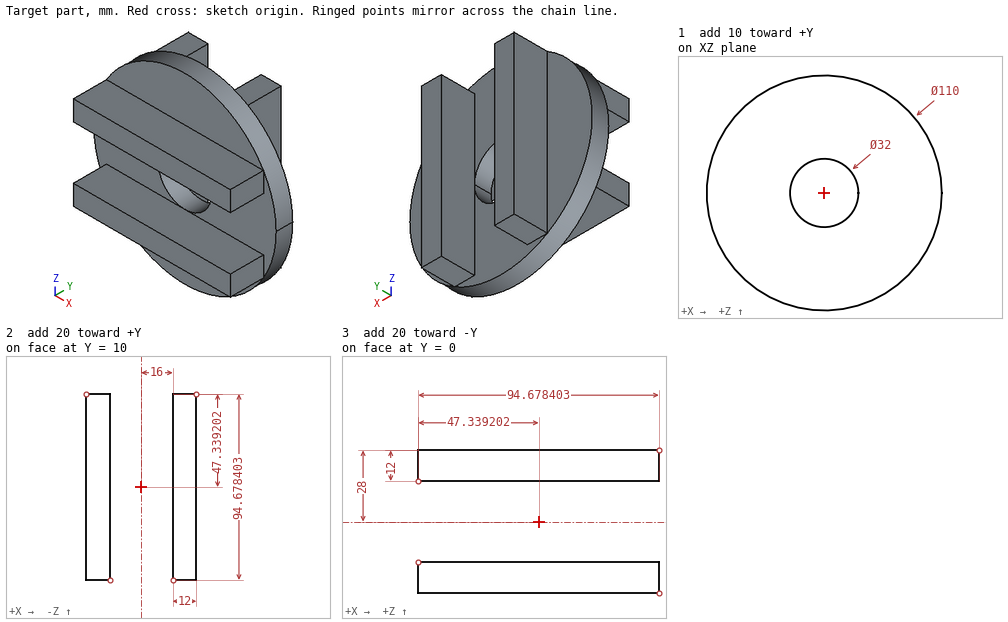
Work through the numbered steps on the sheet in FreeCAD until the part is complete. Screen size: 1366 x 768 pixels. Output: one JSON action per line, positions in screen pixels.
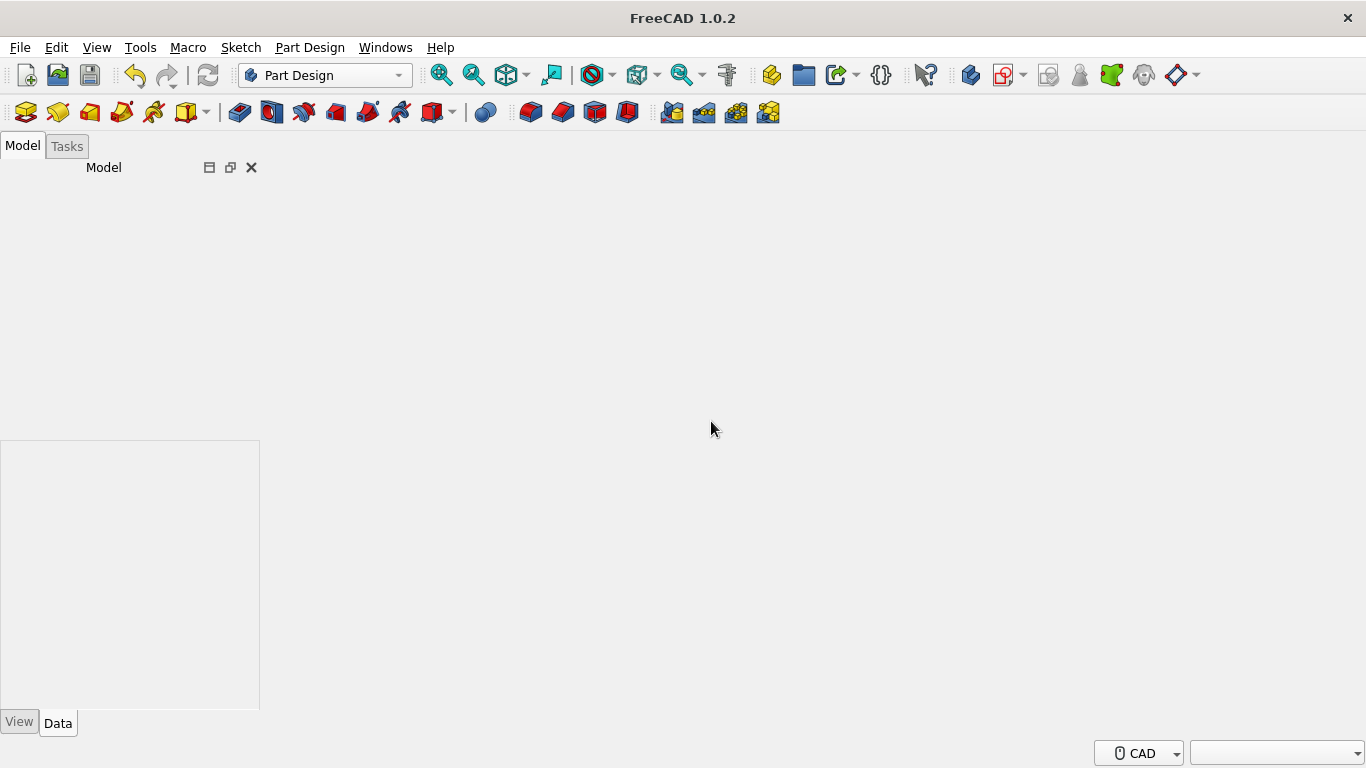
{"action": "left_click", "coordinate": [26, 76]}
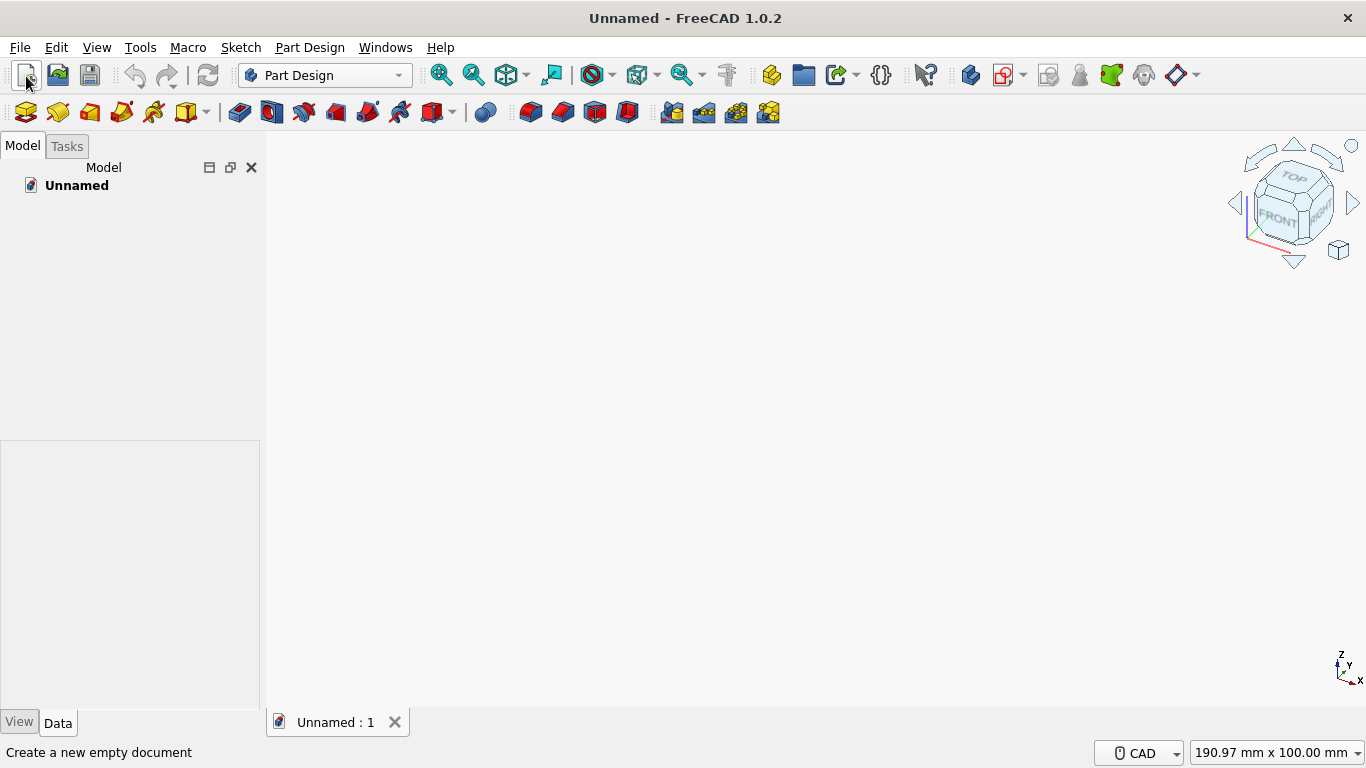
{"action": "left_click", "coordinate": [1004, 76]}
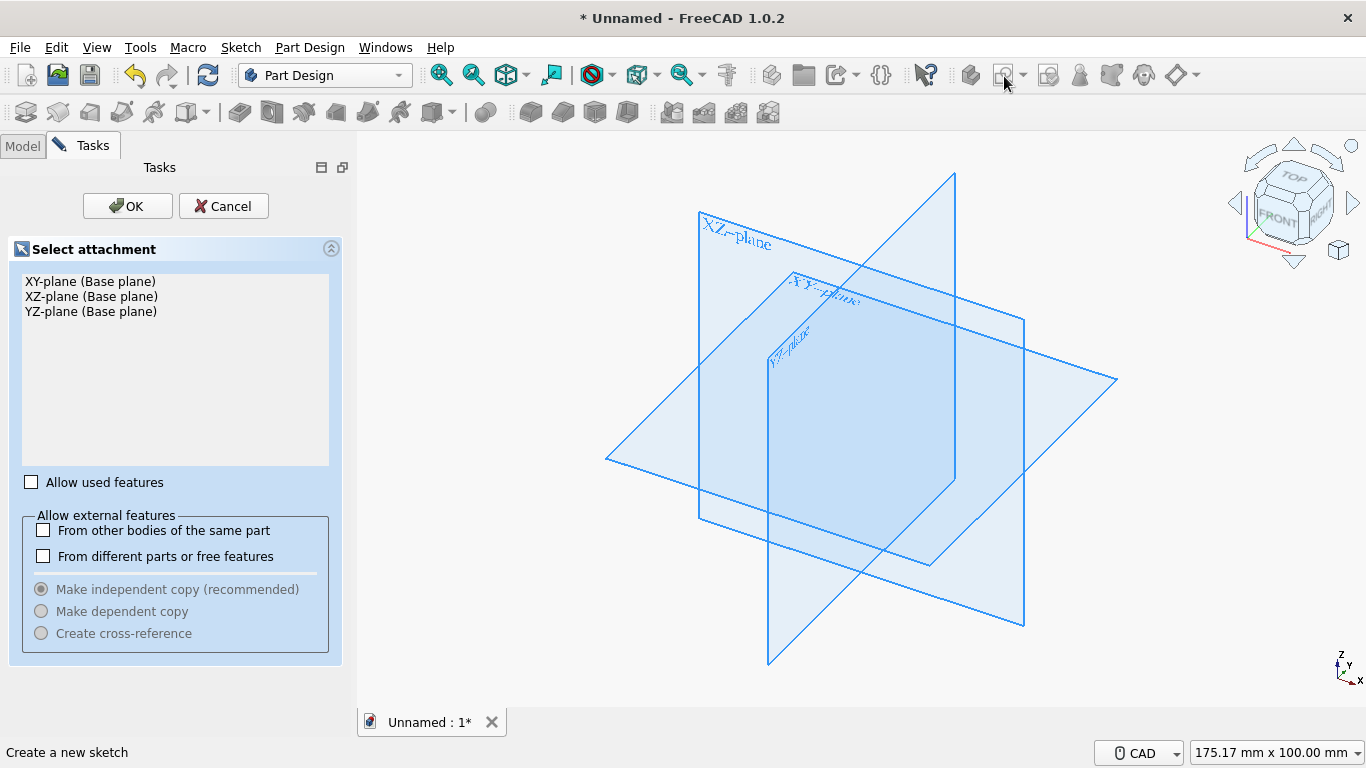
{"action": "left_click", "coordinate": [82, 296]}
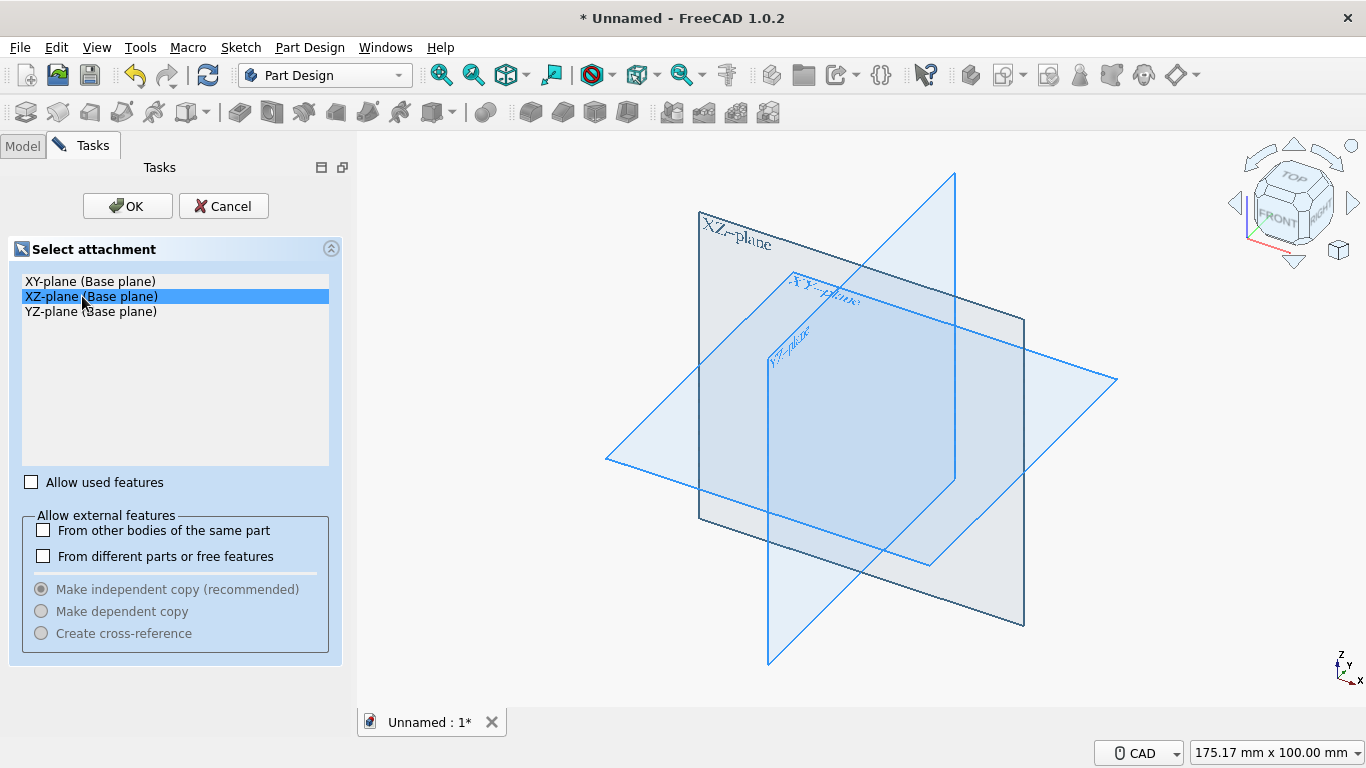
{"action": "left_click", "coordinate": [128, 206]}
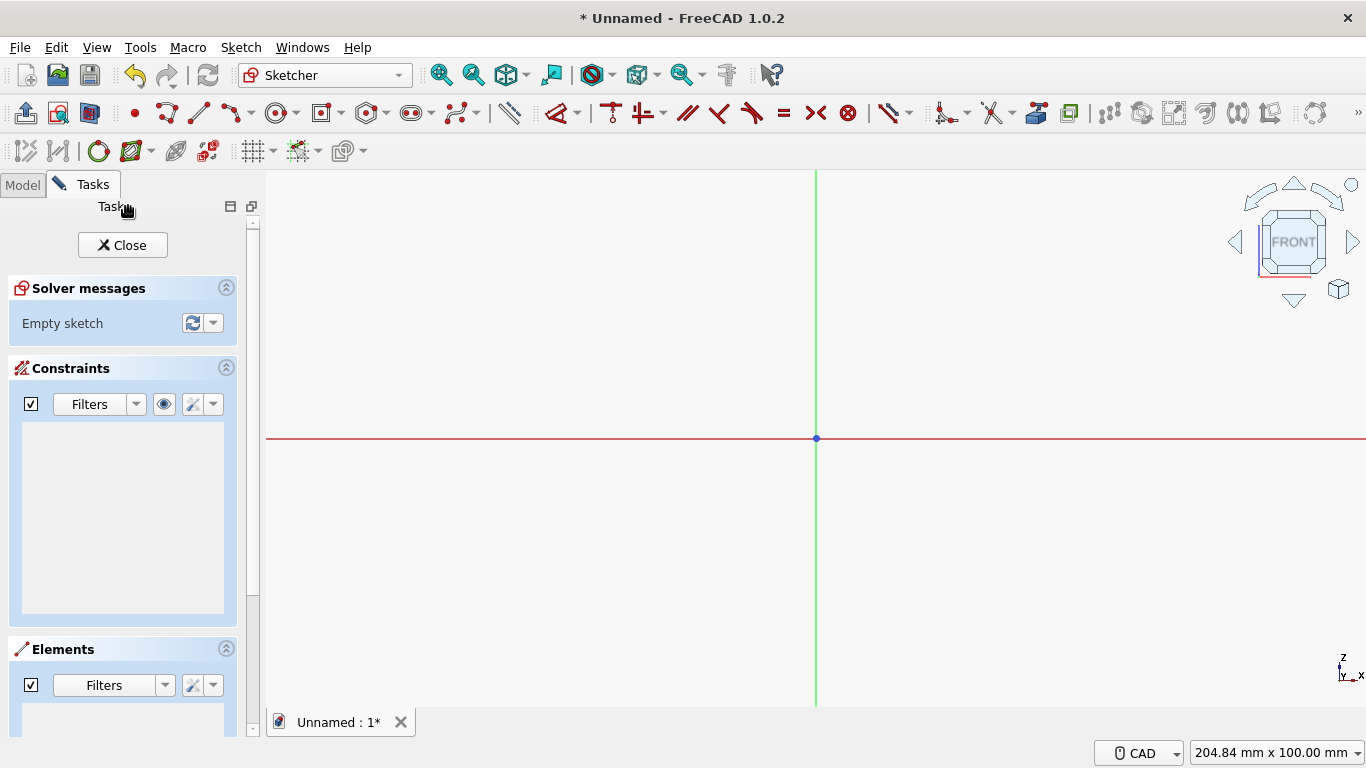
{"action": "scroll", "coordinate": [664, 438], "scroll_direction": "down", "scroll_amount": 3}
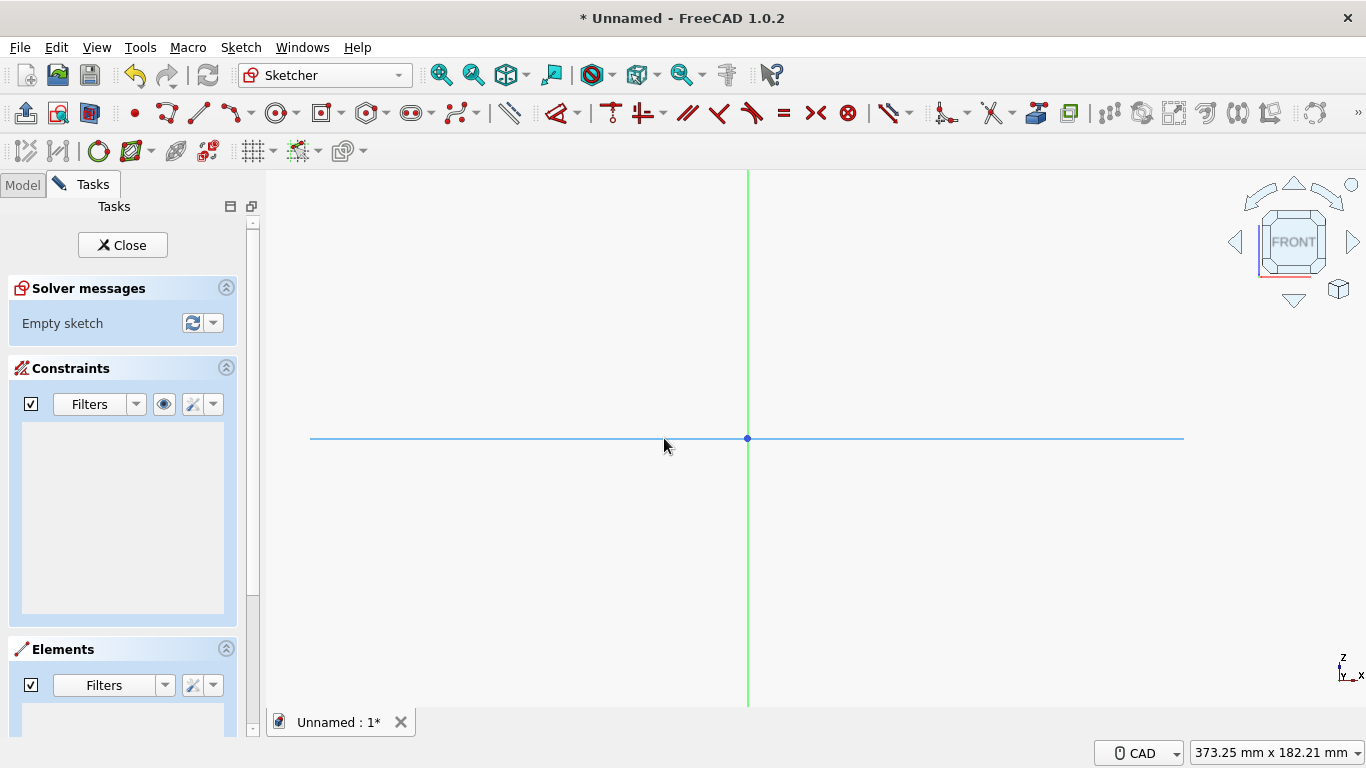
{"action": "key", "text": "g c"}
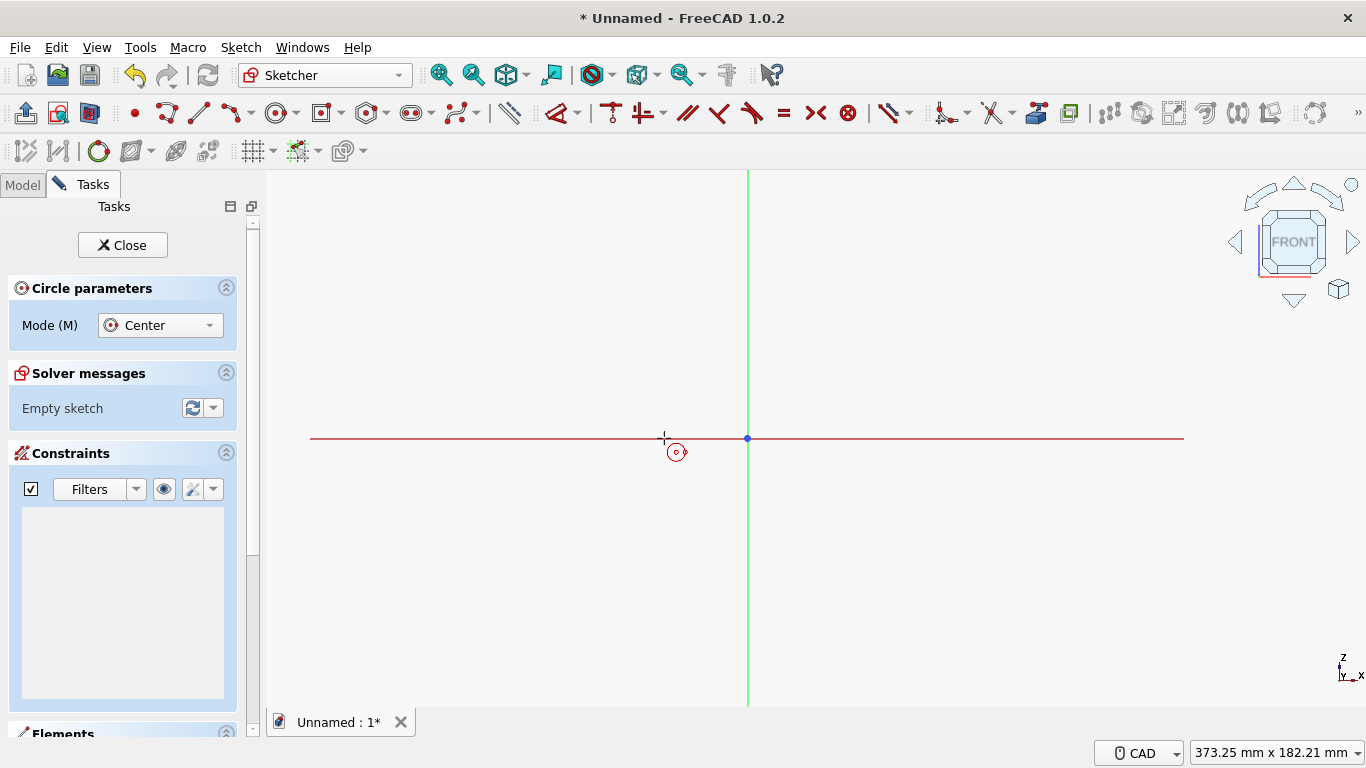
{"action": "left_click", "coordinate": [748, 438]}
{"action": "left_click", "coordinate": [862, 324]}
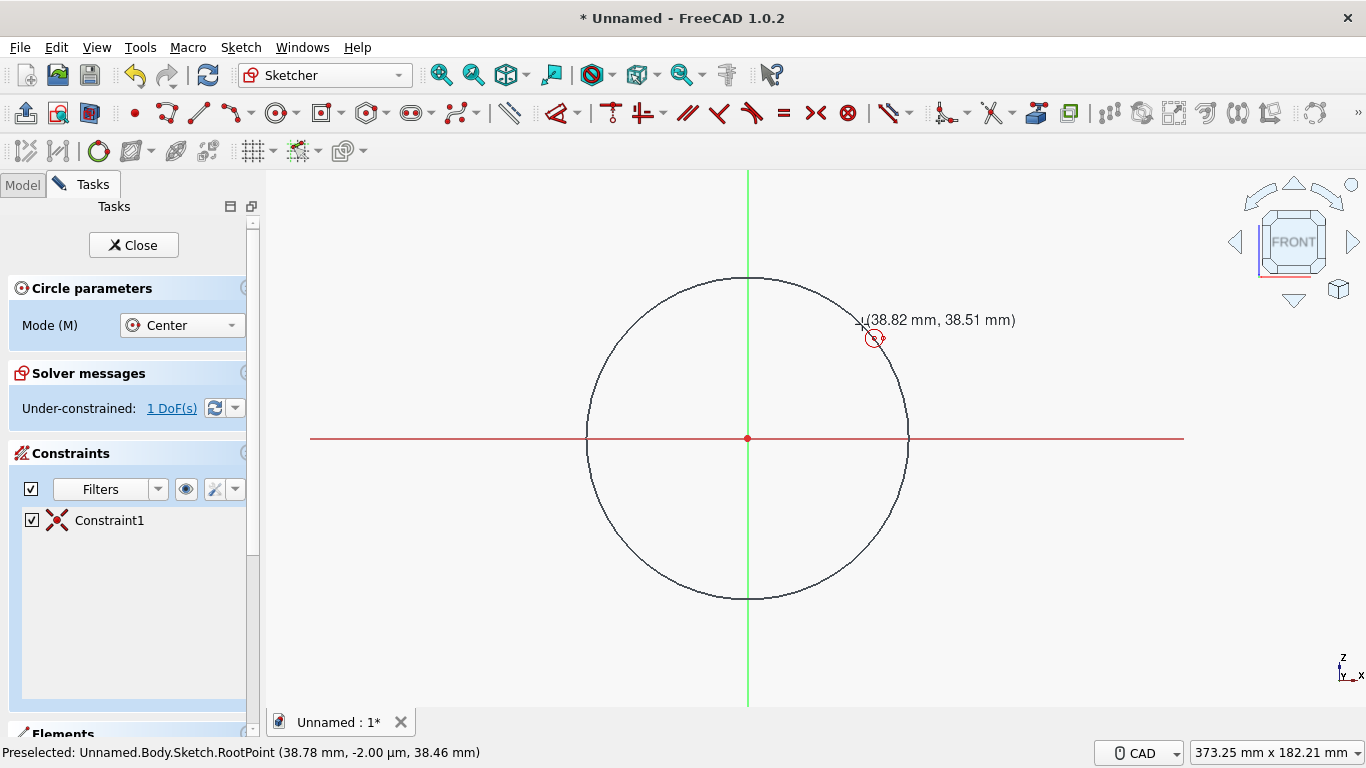
{"action": "left_click", "coordinate": [748, 438]}
{"action": "left_click", "coordinate": [781, 405]}
{"action": "key", "text": "Escape"}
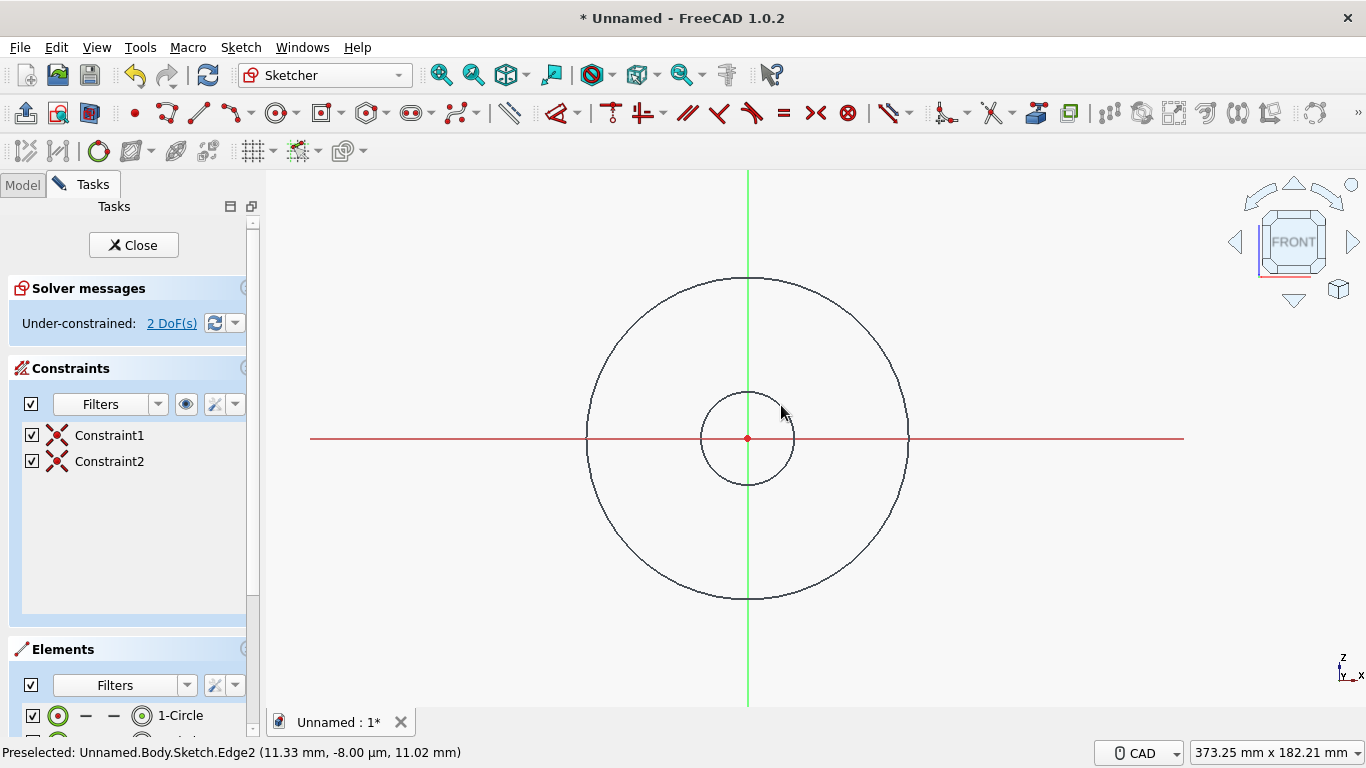
{"action": "left_click", "coordinate": [861, 324]}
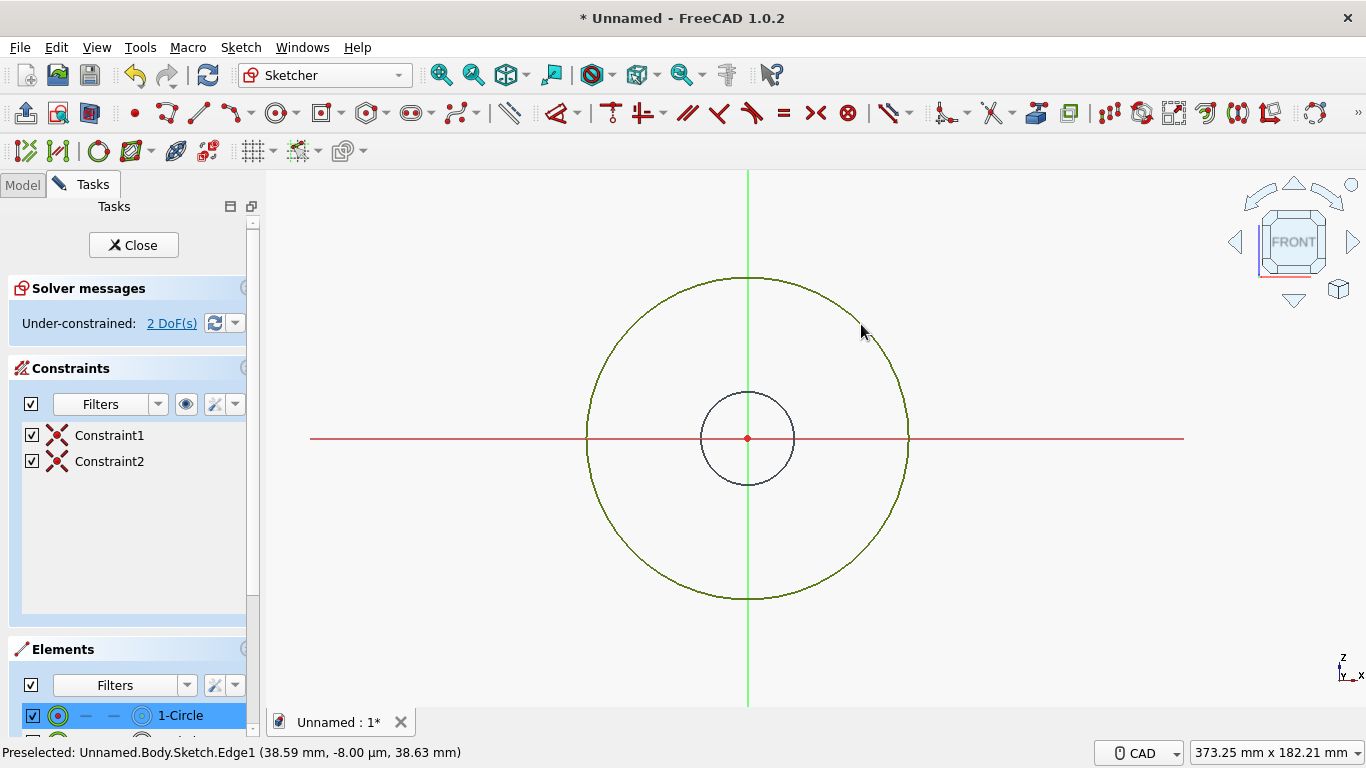
{"action": "key", "text": "k o"}